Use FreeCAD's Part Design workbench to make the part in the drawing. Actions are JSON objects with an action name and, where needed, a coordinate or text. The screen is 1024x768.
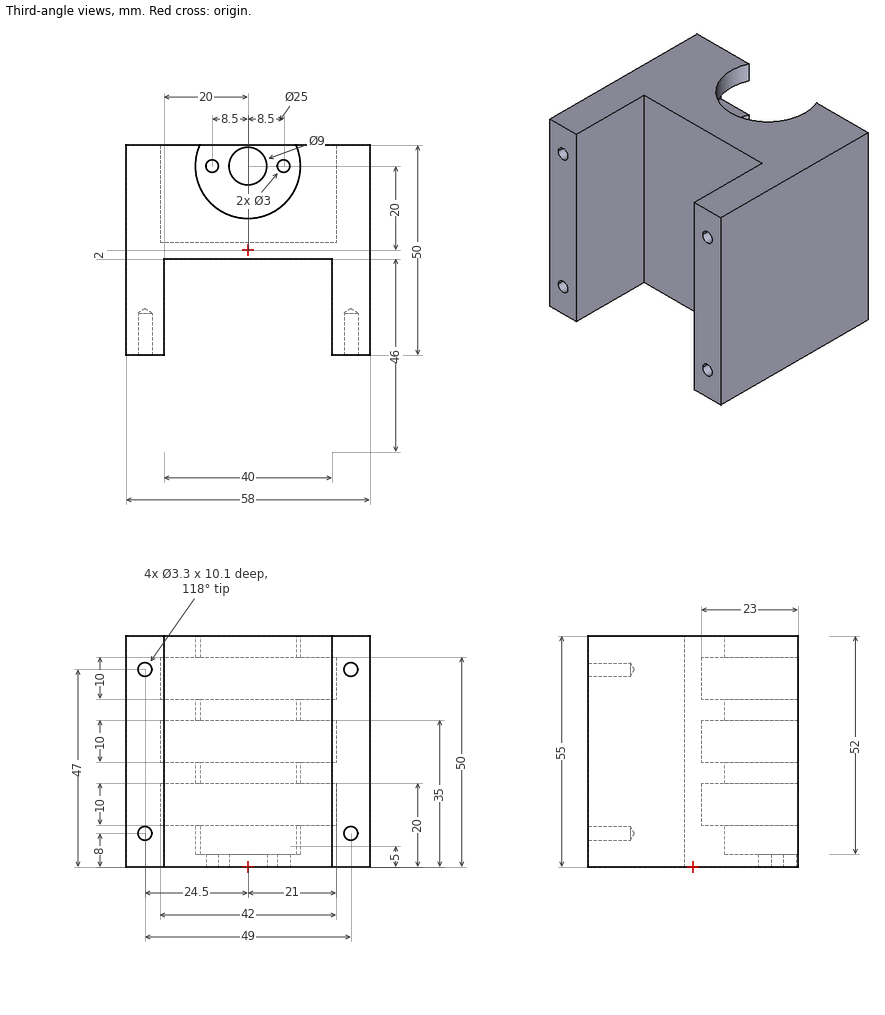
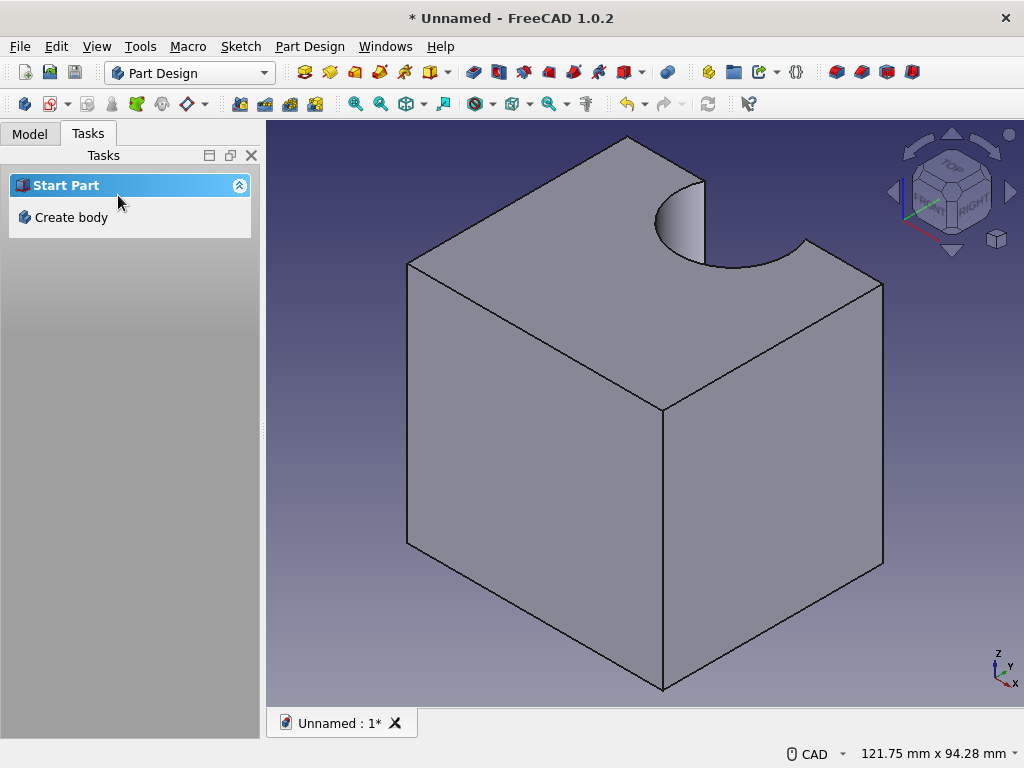
{"action": "left_click", "coordinate": [50, 104]}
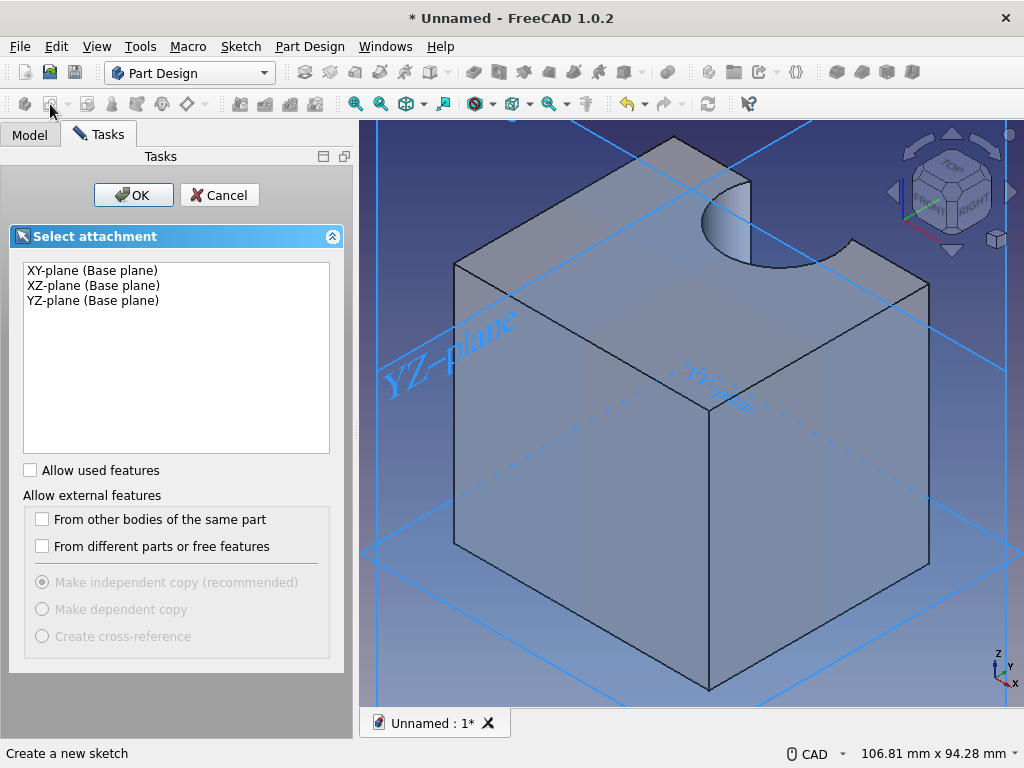
{"action": "left_click", "coordinate": [84, 270]}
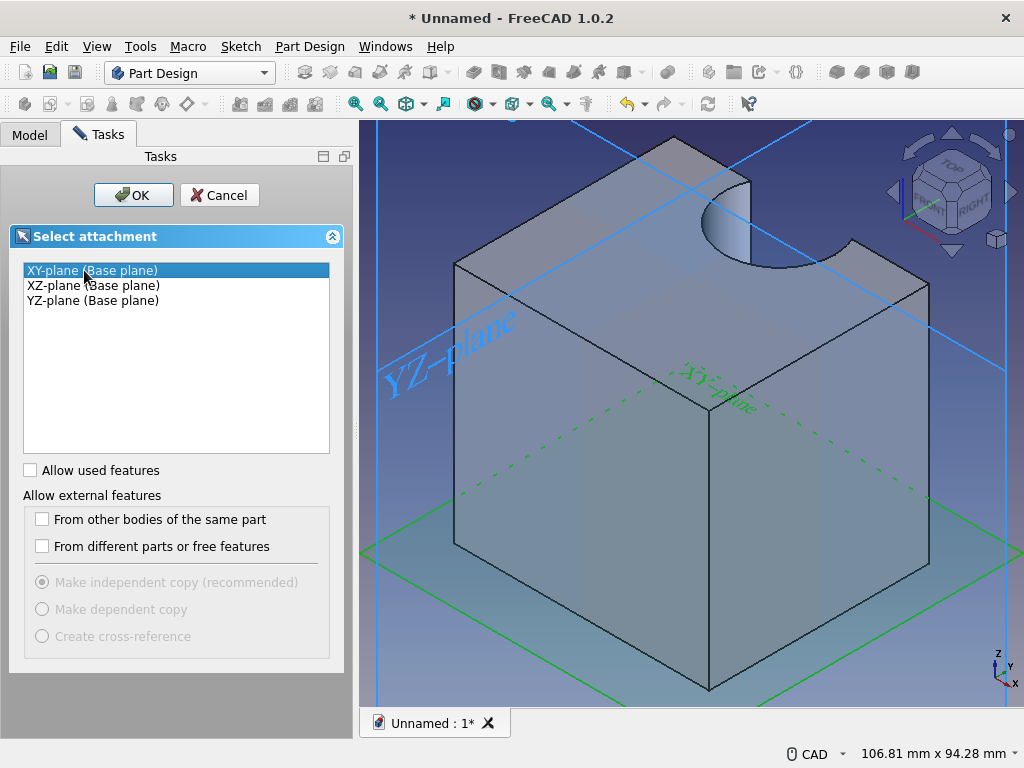
{"action": "left_click", "coordinate": [134, 195]}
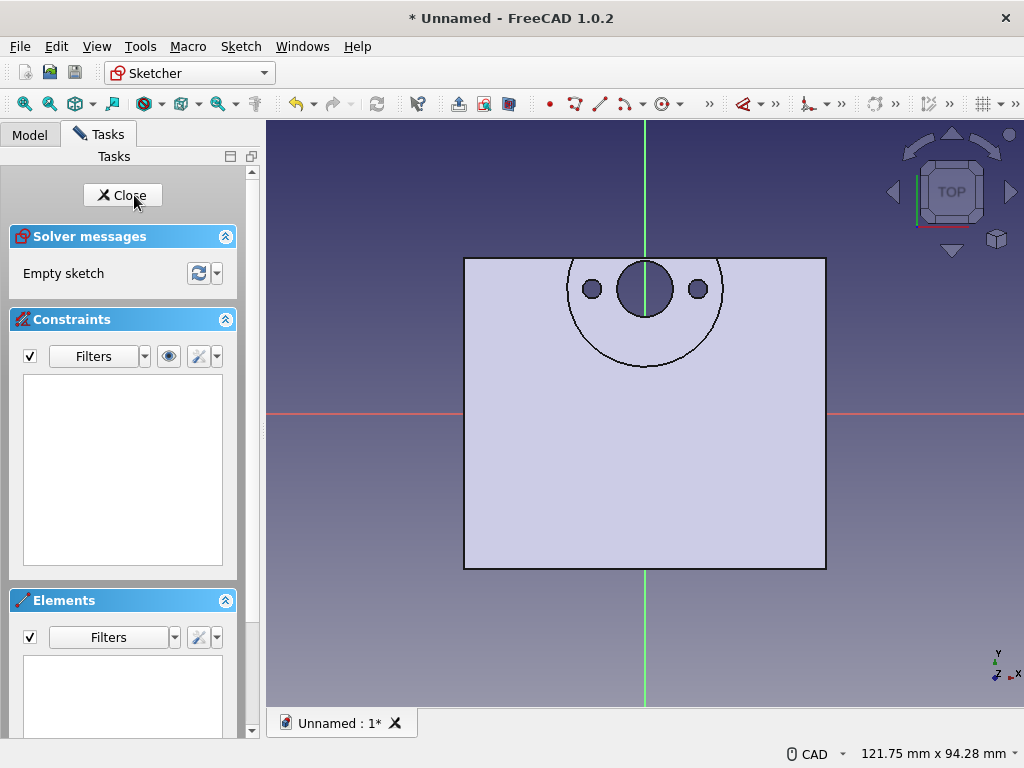
{"action": "left_click", "coordinate": [509, 104]}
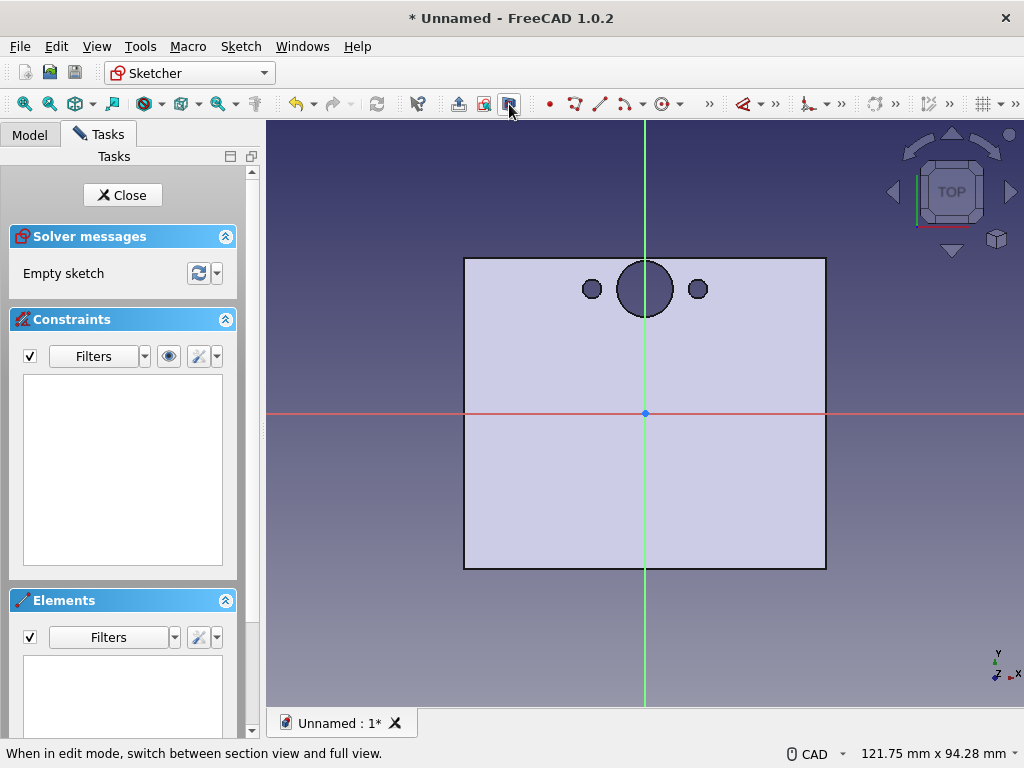
{"action": "scroll", "coordinate": [294, 148], "scroll_direction": "down", "scroll_amount": 1}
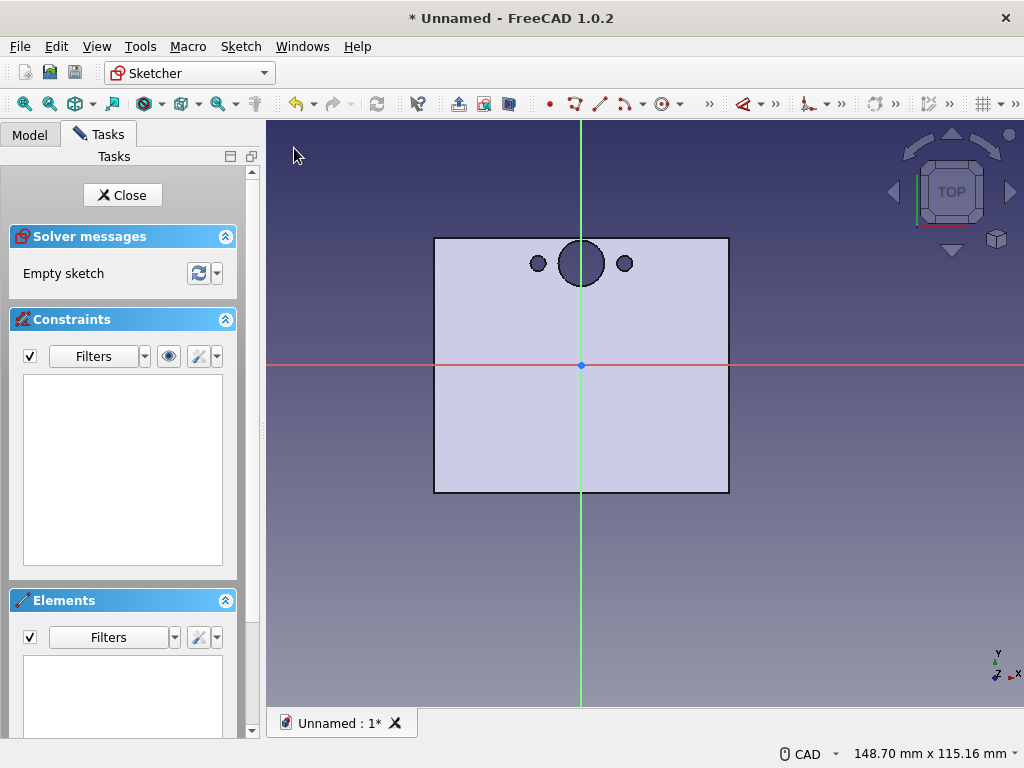
{"action": "scroll", "coordinate": [591, 639], "scroll_direction": "up", "scroll_amount": 2}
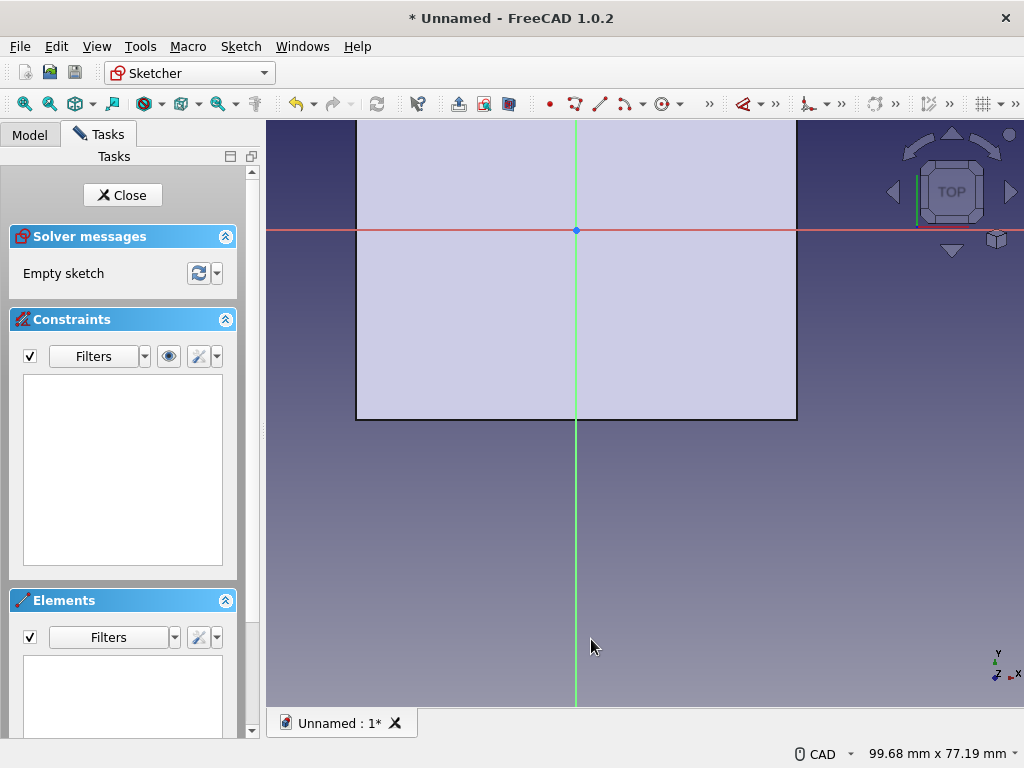
{"action": "key", "text": "g r"}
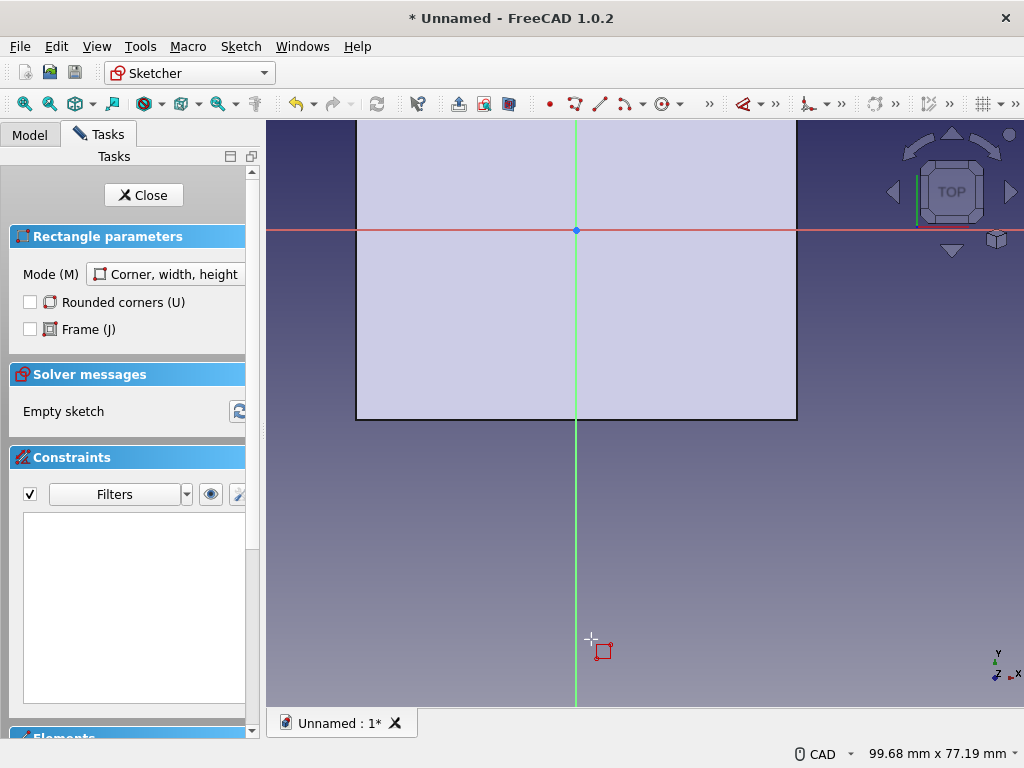
{"action": "left_click", "coordinate": [424, 246]}
{"action": "mouse_move", "coordinate": [729, 595]}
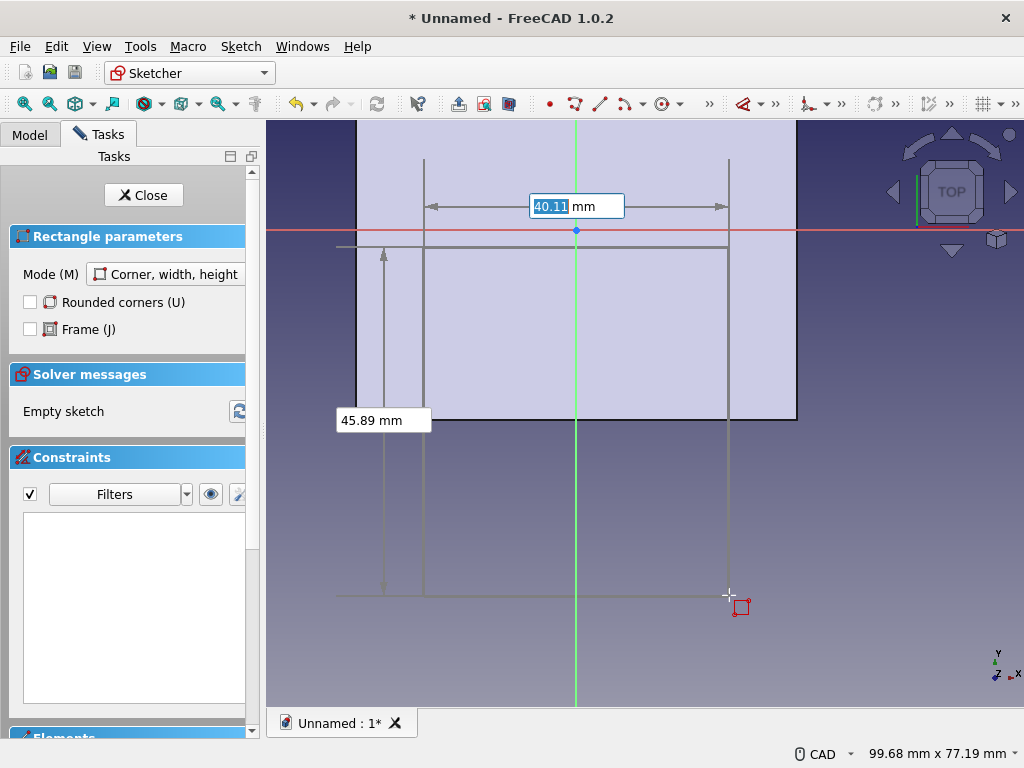
{"action": "type", "text": "40"}
{"action": "key", "text": "Tab"}
{"action": "type", "text": "46"}
{"action": "key", "text": "Return"}
{"action": "key", "text": "Escape"}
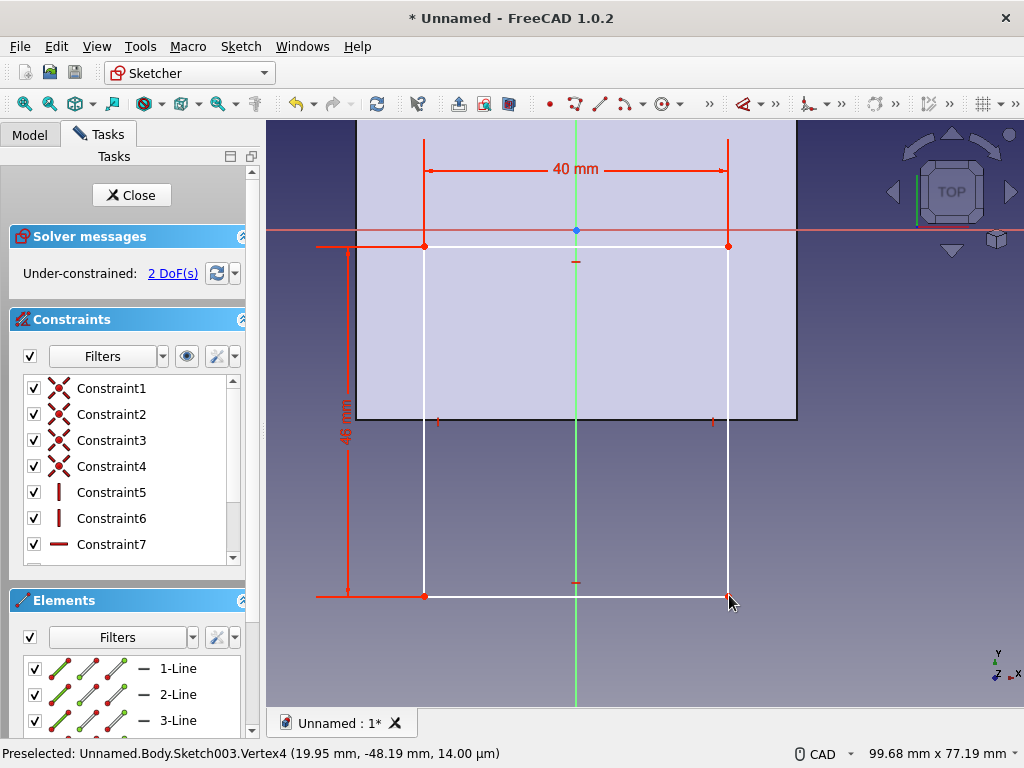
{"action": "key", "text": "d"}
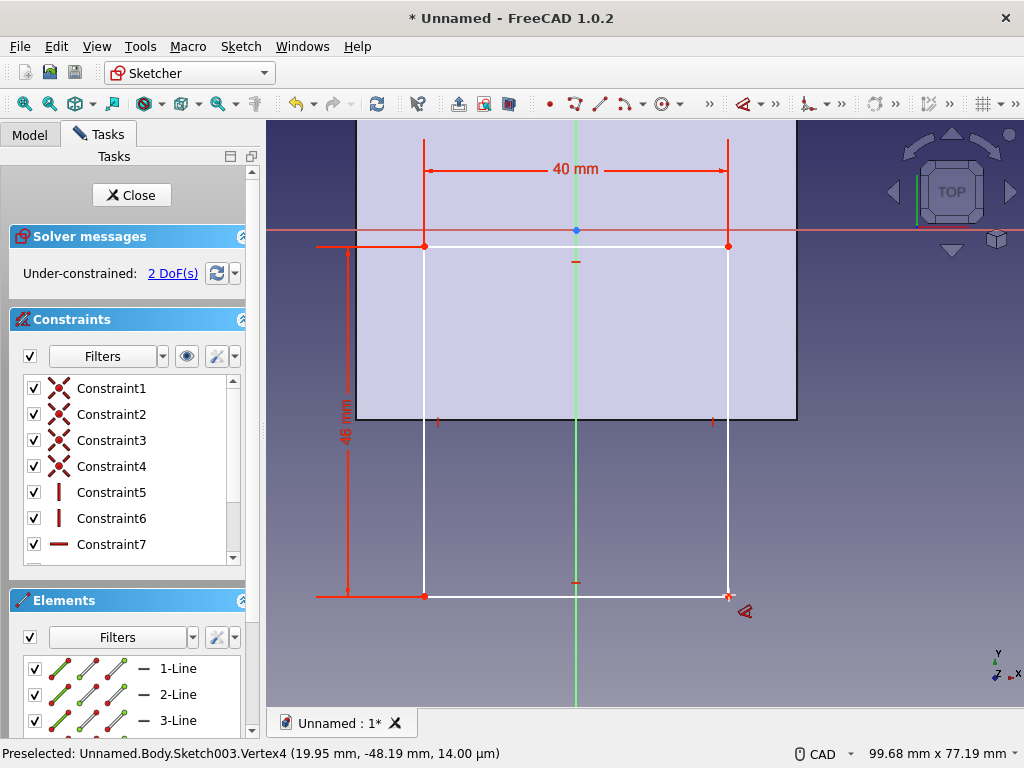
{"action": "scroll", "coordinate": [424, 247], "scroll_direction": "up", "scroll_amount": 5}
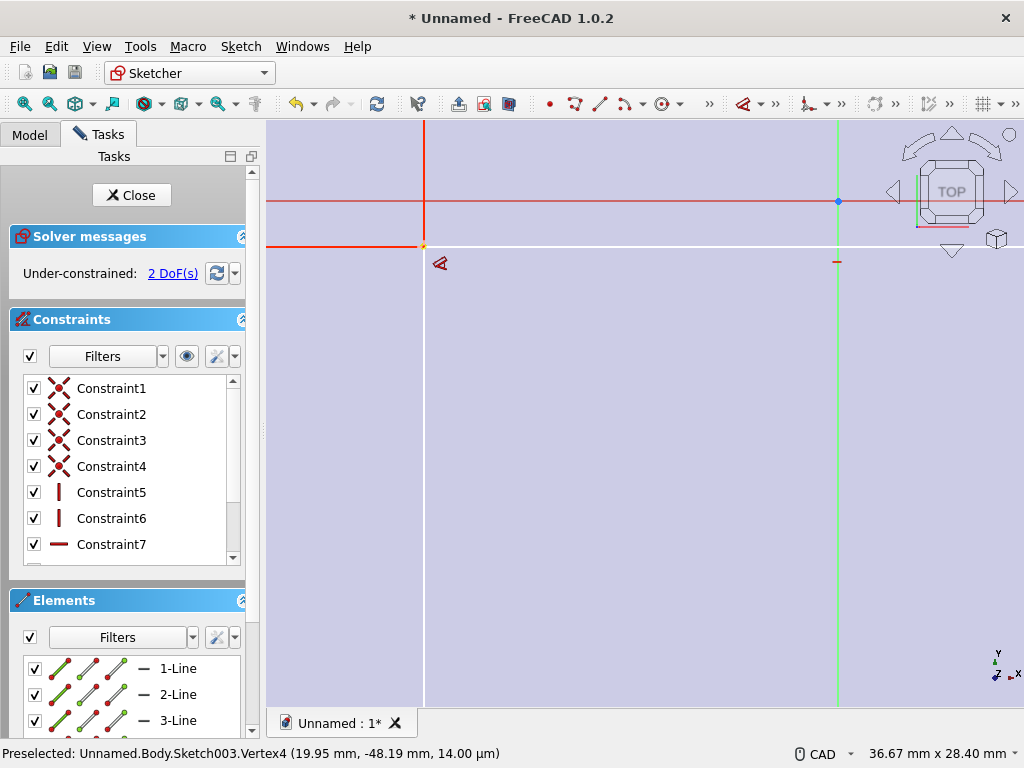
{"action": "left_click", "coordinate": [424, 247]}
{"action": "left_click", "coordinate": [390, 224]}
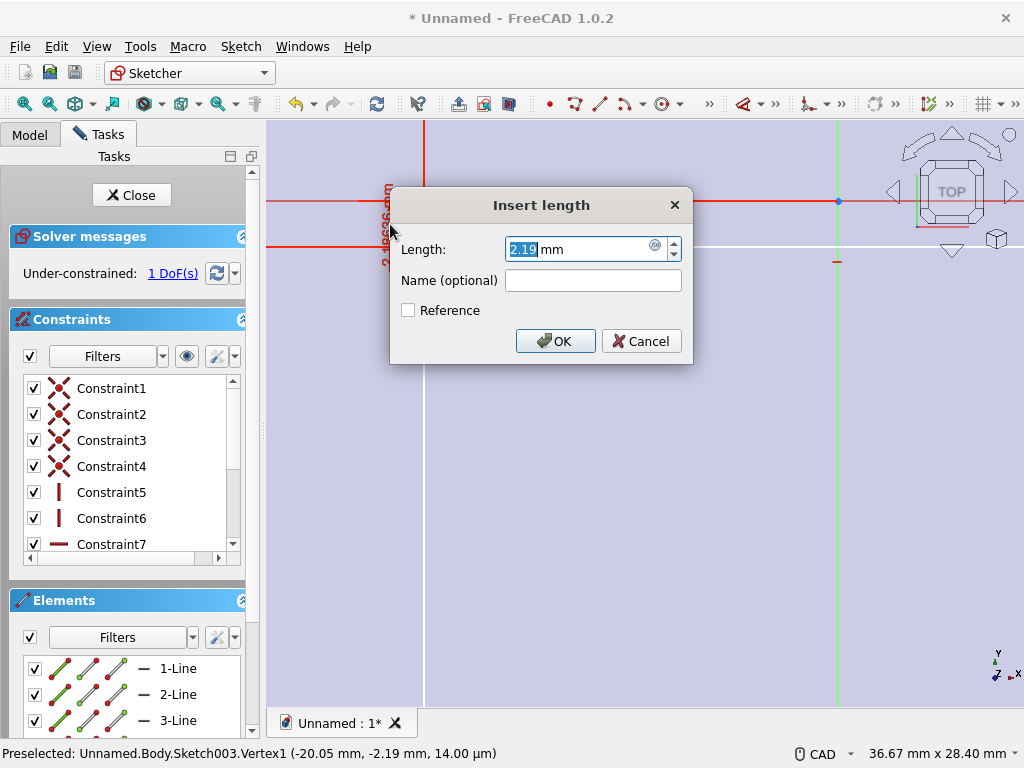
{"action": "type", "text": "2"}
{"action": "key", "text": "Return"}